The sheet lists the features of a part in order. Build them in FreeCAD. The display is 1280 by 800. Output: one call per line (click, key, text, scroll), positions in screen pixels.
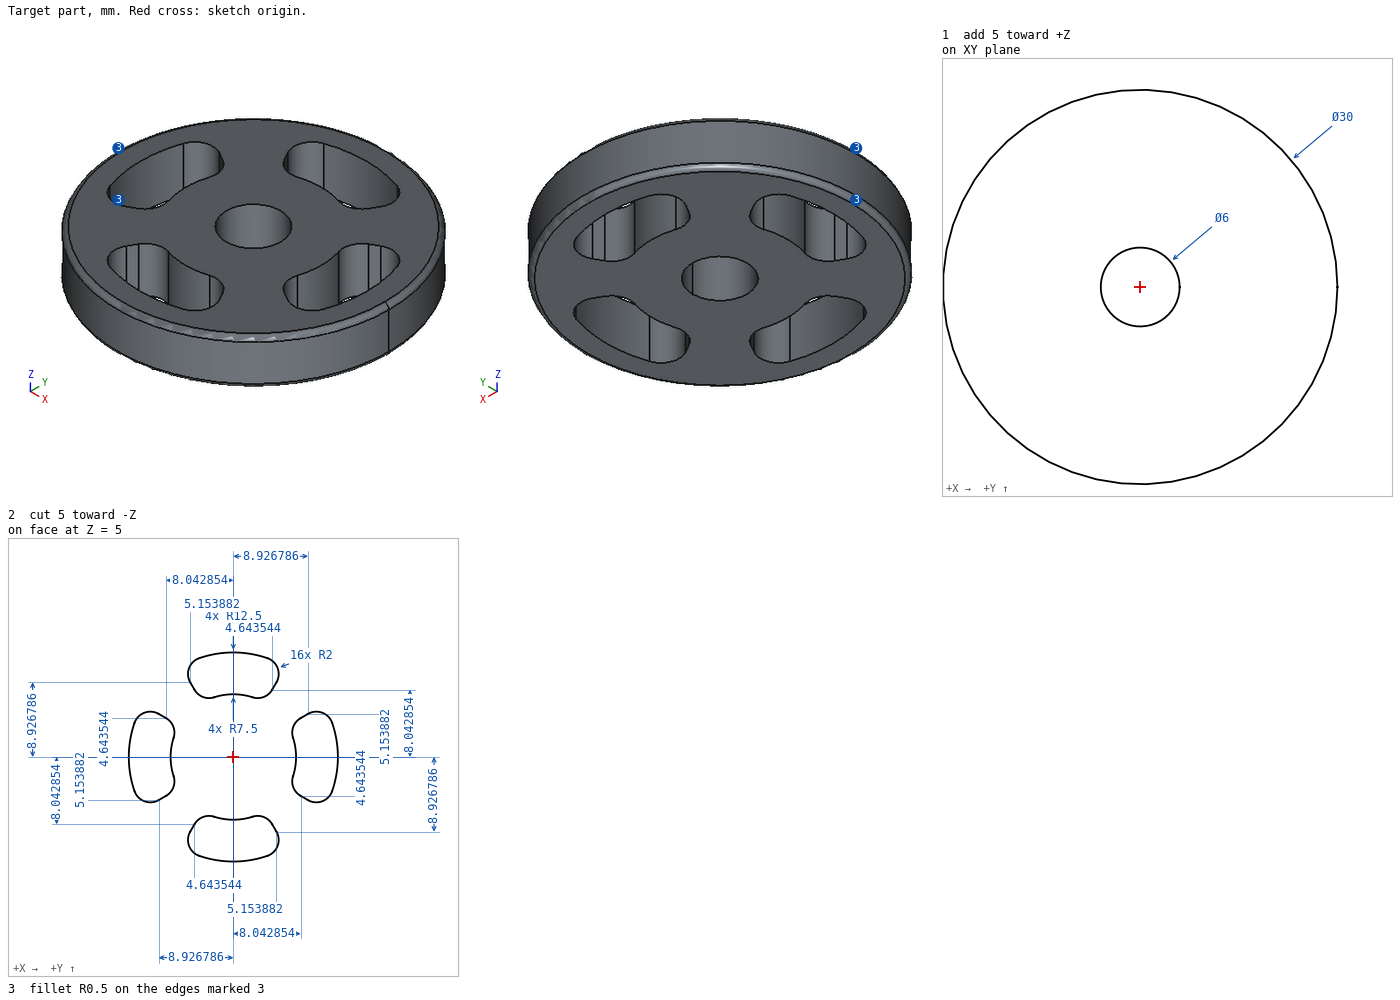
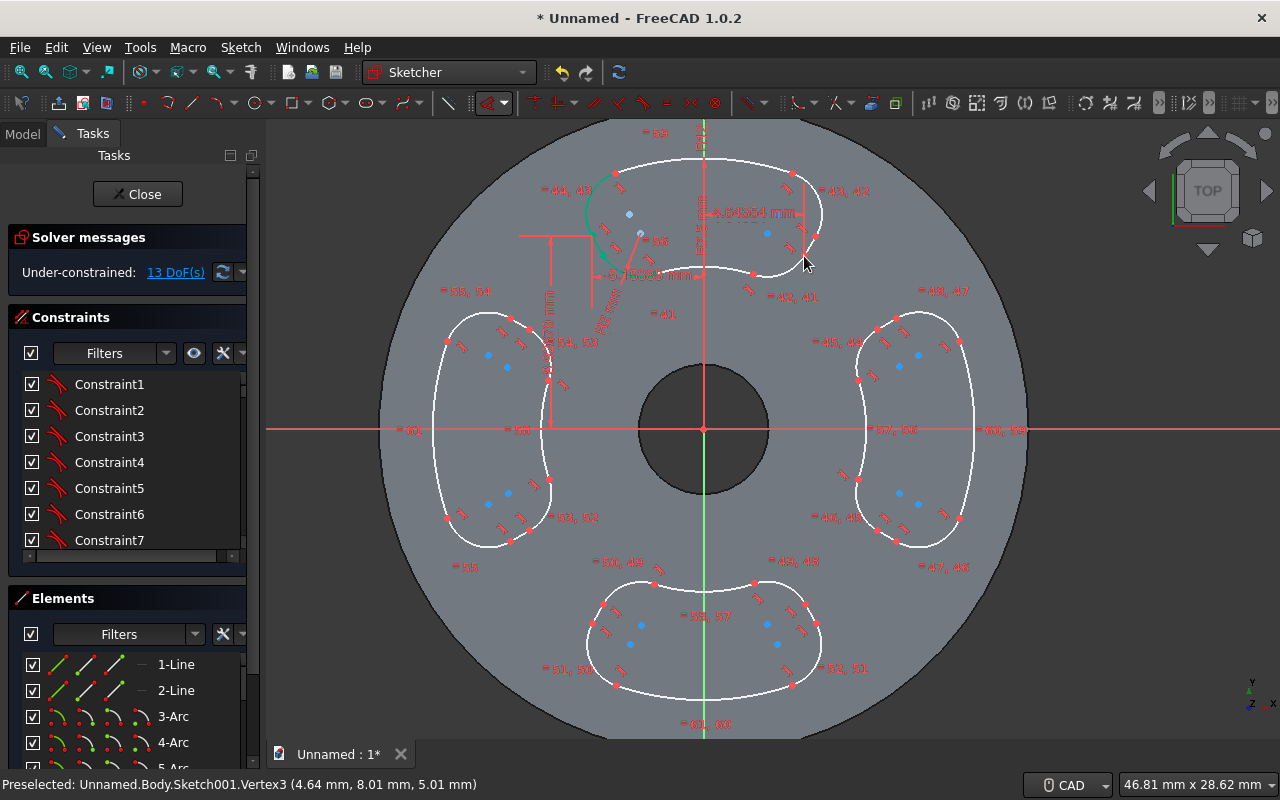
click(804, 256)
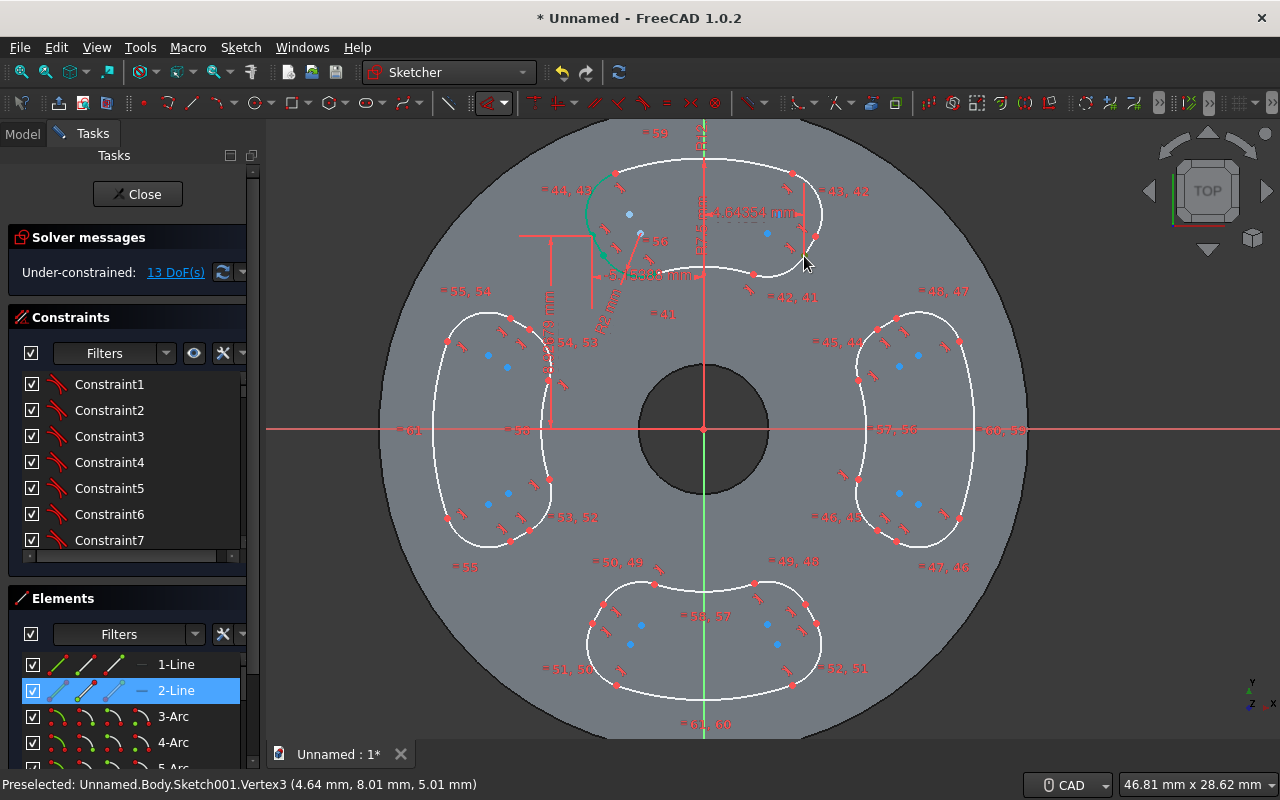
click(506, 104)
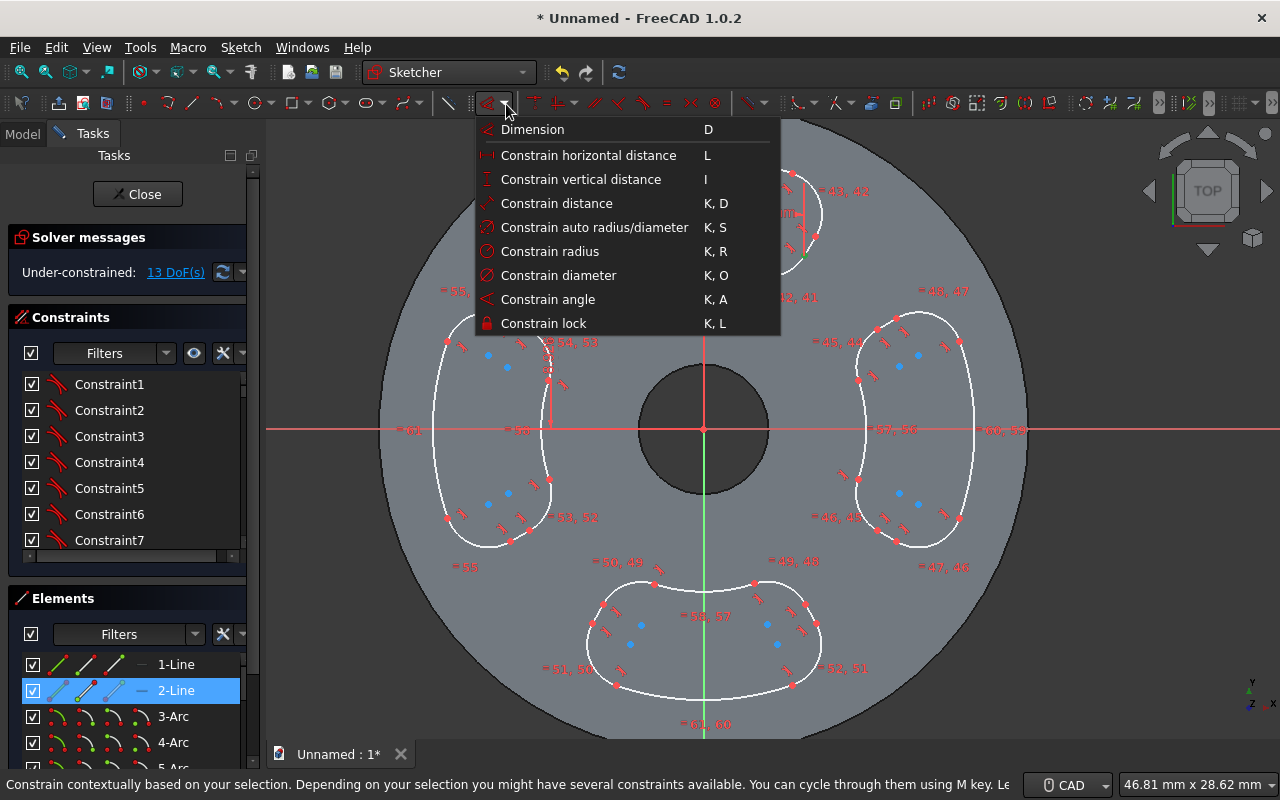
click(628, 179)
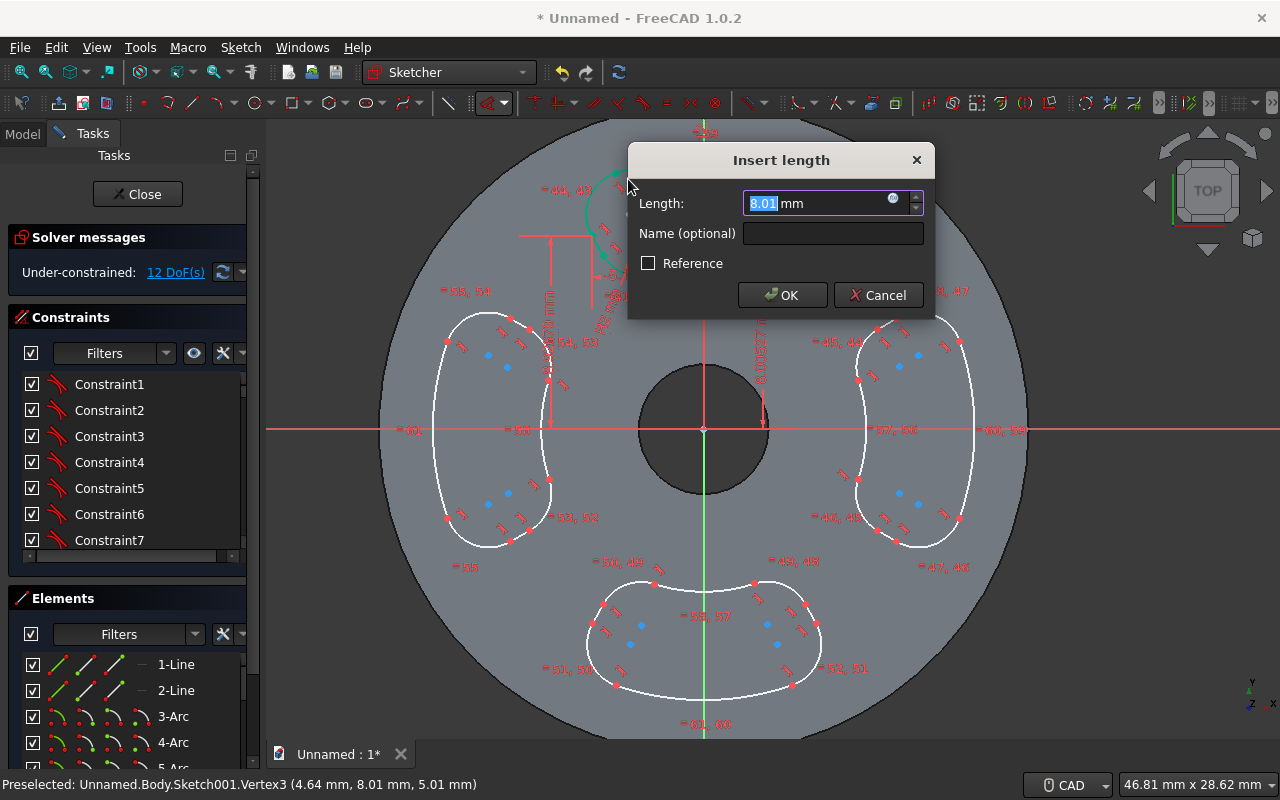
text(8.042854)
key(Return)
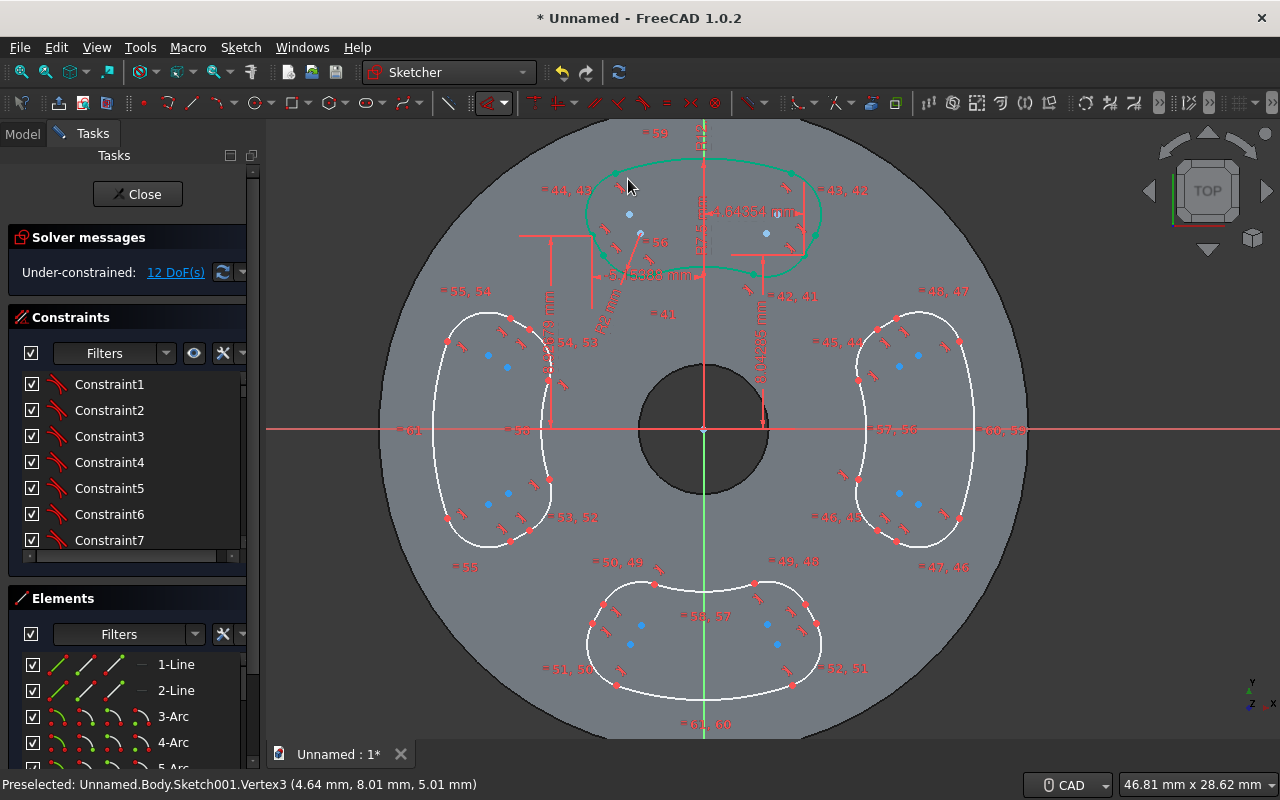
click(897, 318)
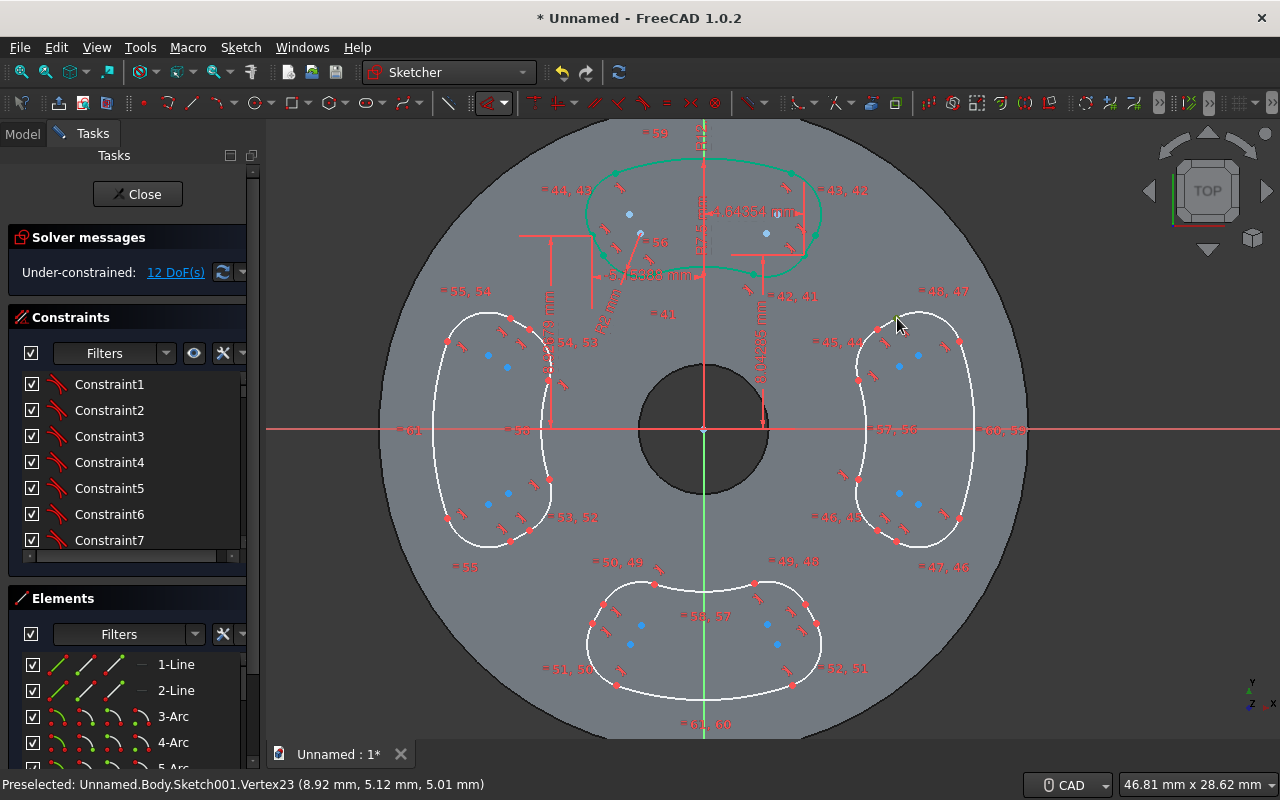
key(l)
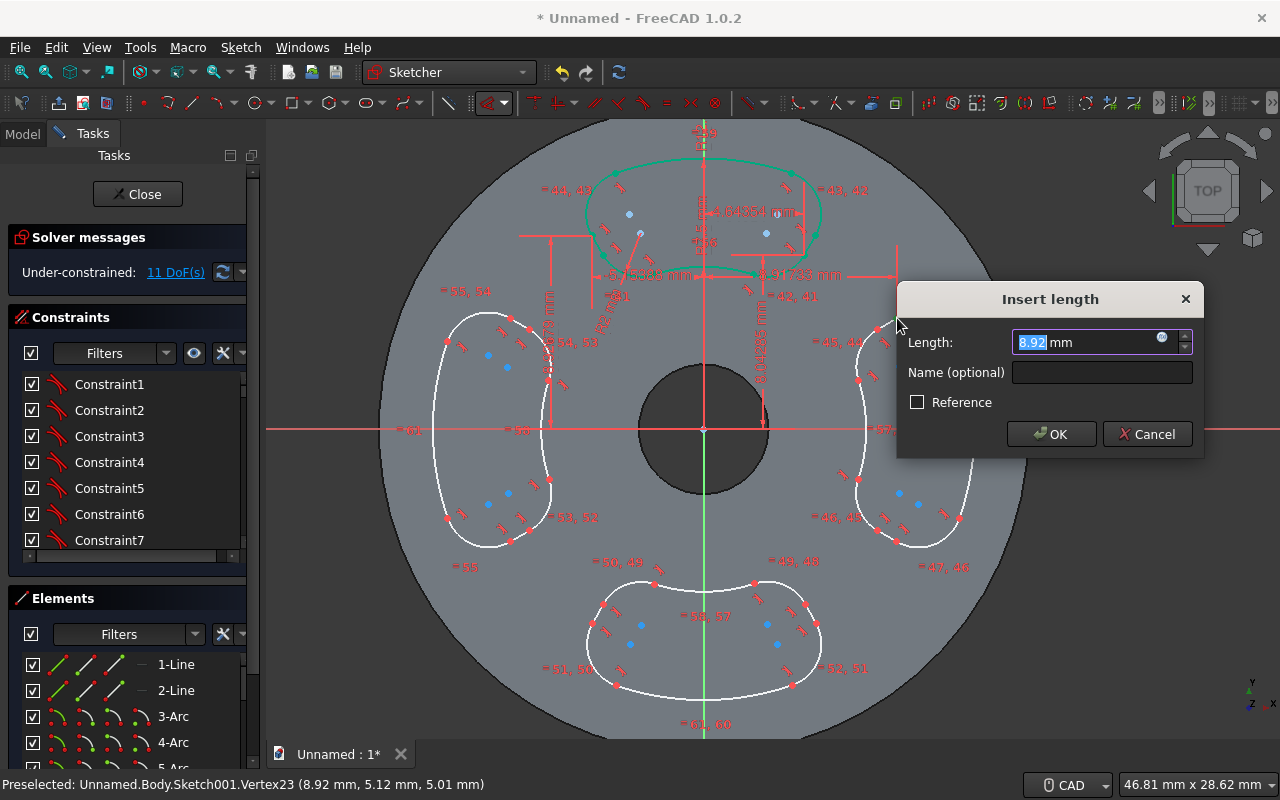
text(8.926786)
key(Return)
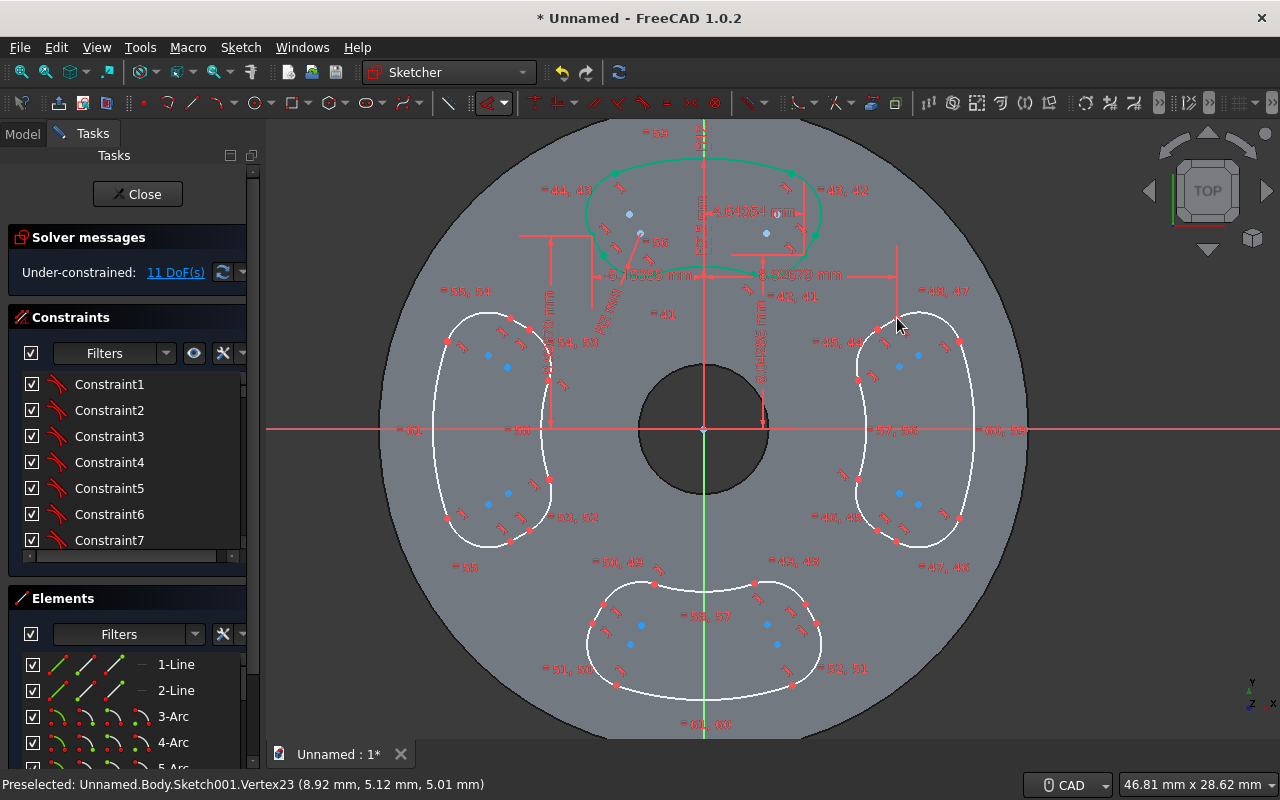
click(897, 318)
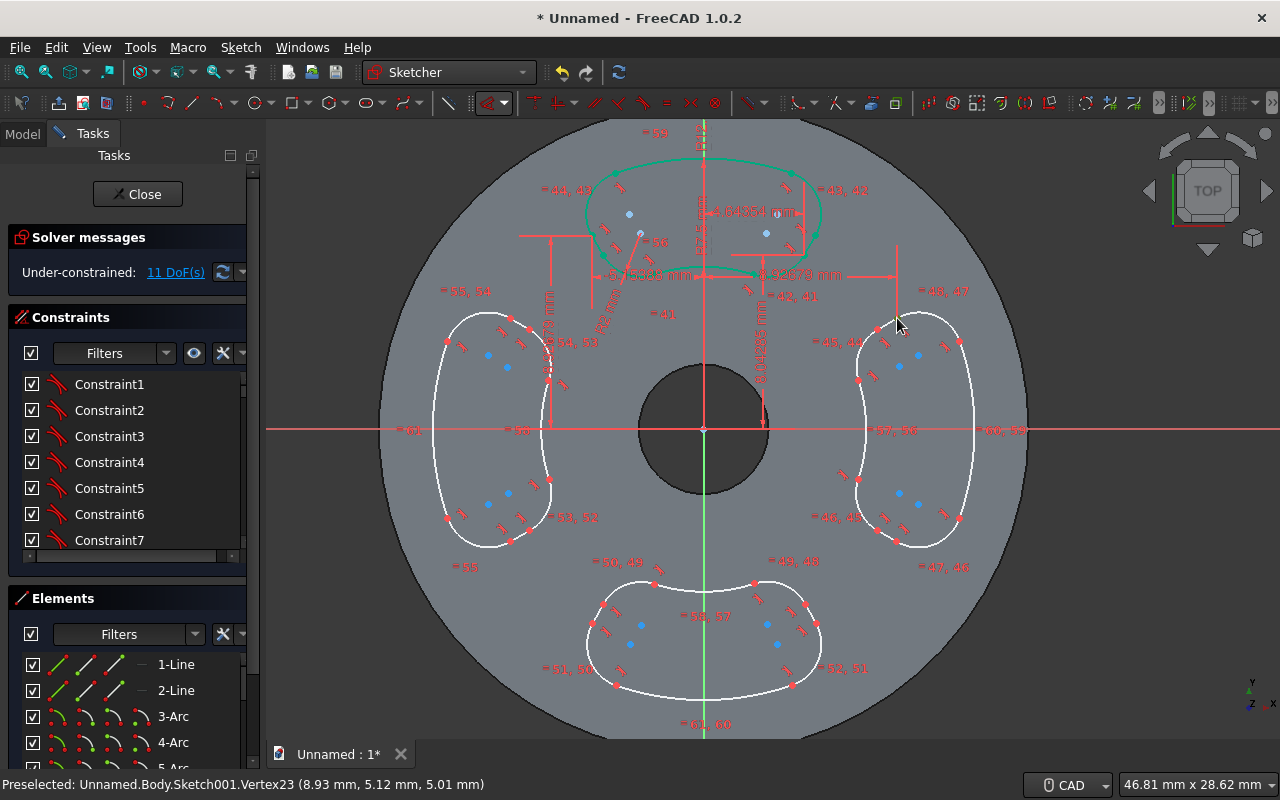
key(i)